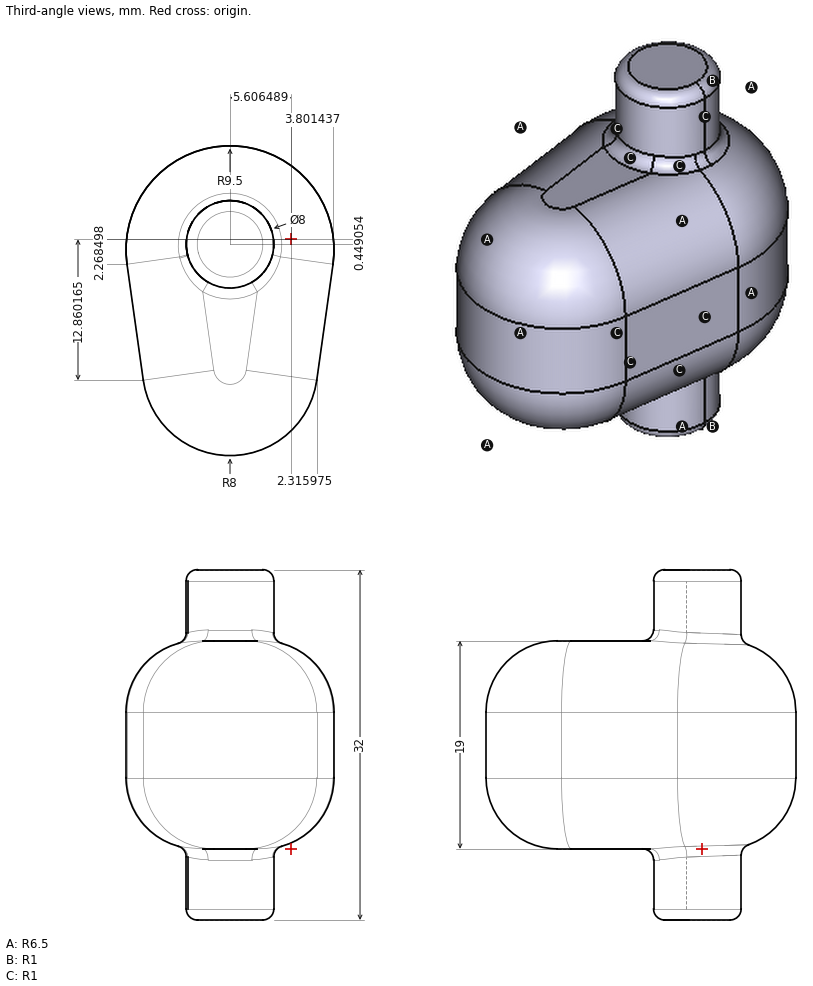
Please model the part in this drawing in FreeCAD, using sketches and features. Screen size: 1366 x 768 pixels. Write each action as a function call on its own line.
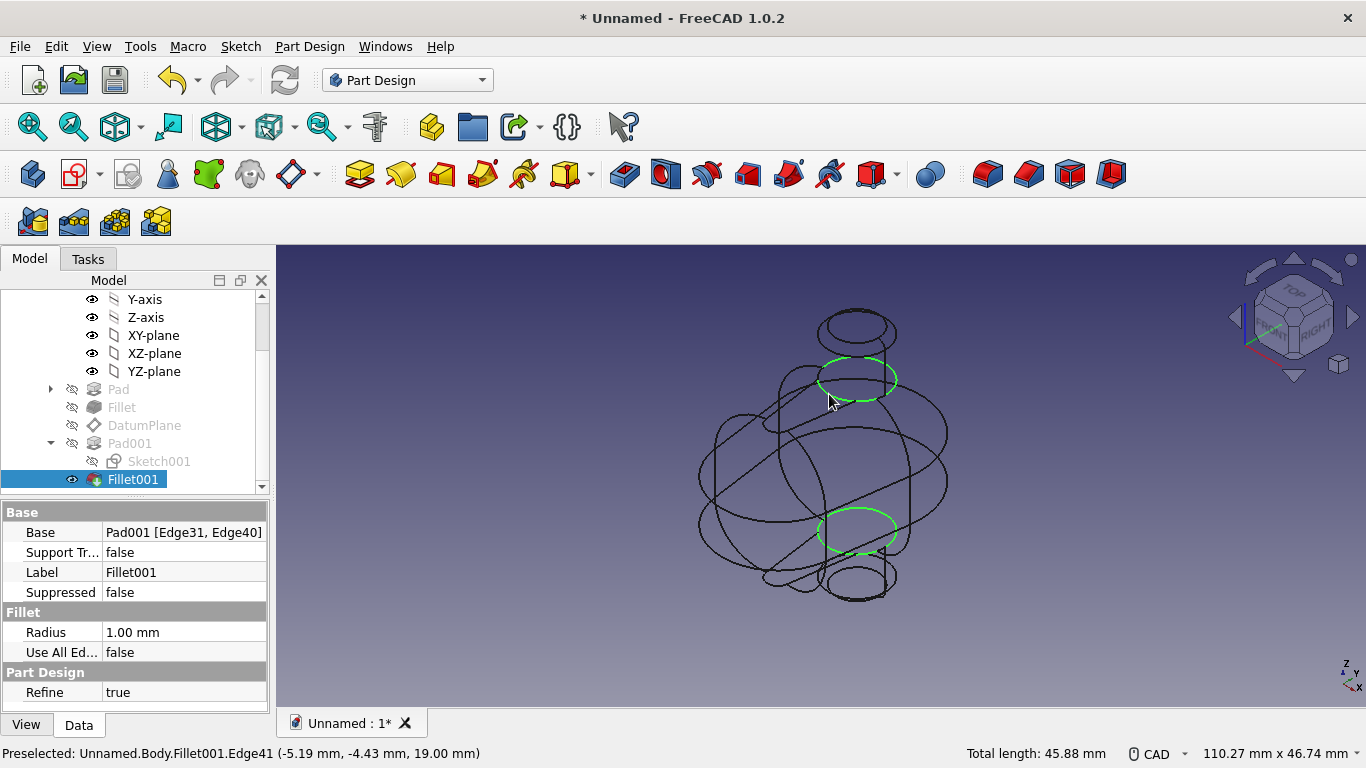
click(819, 372, ctrl)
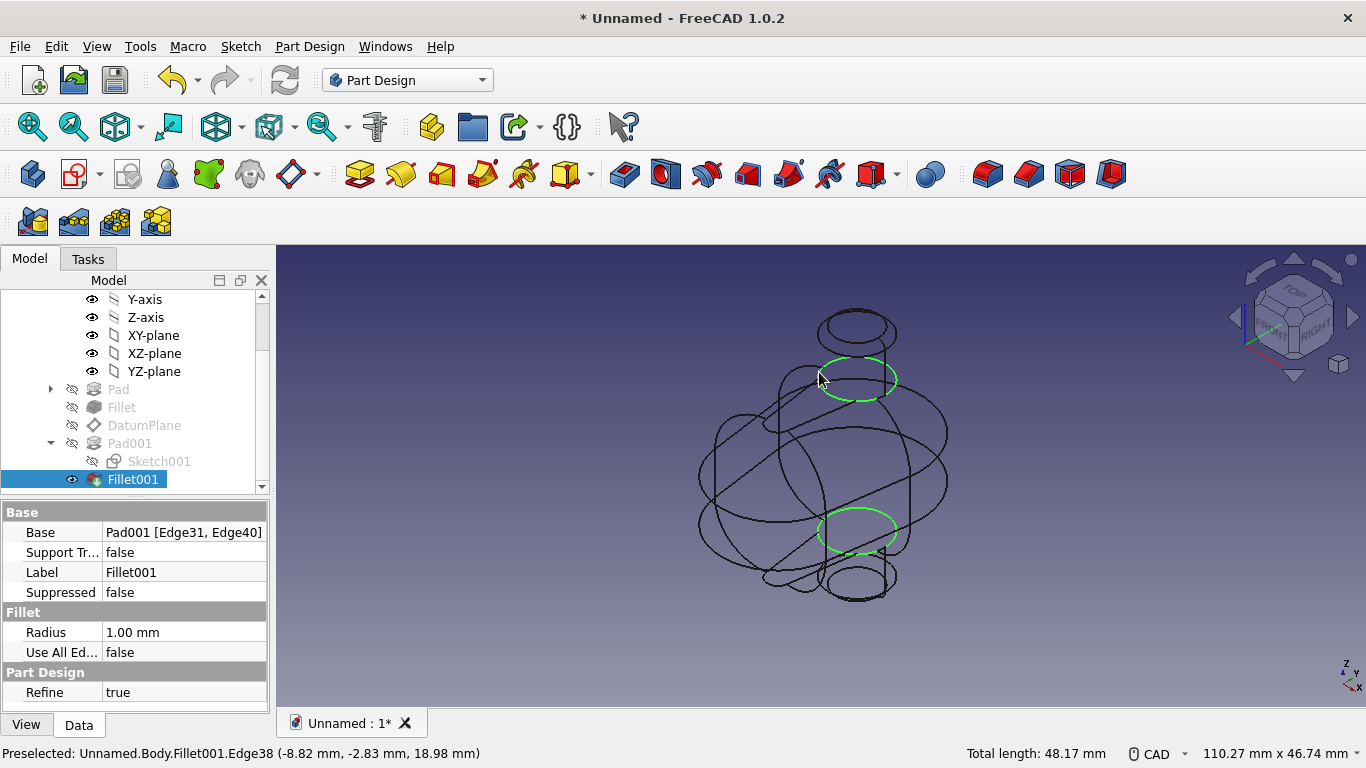
key(v)
key(1)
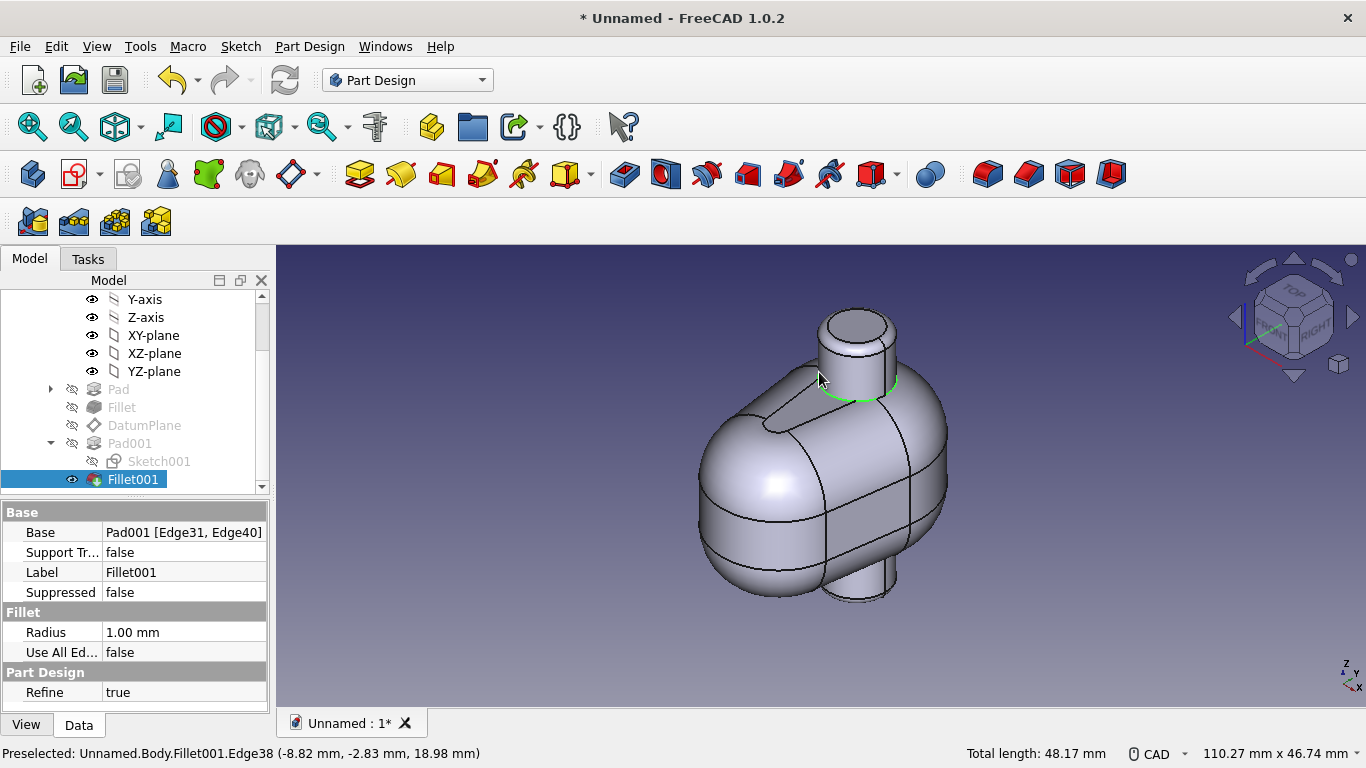
click(988, 174)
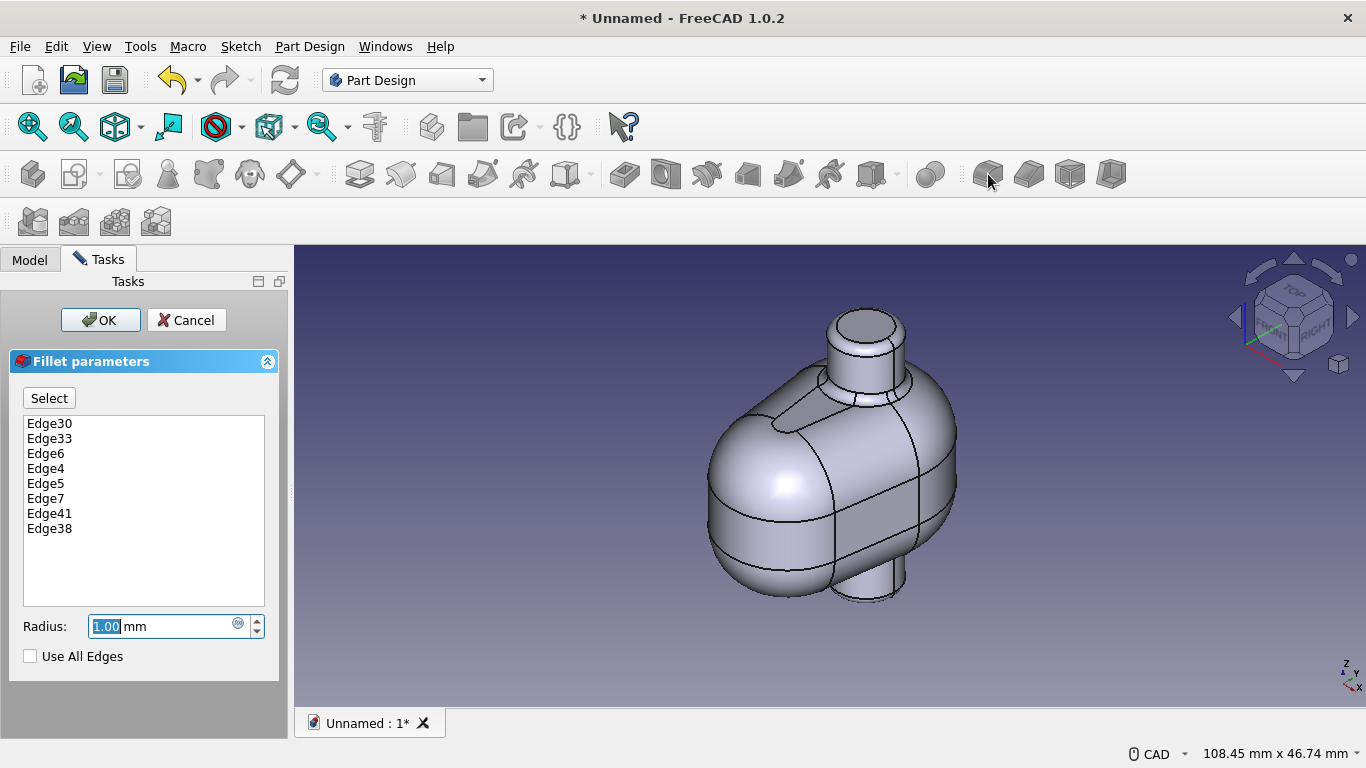
text(1)
key(Tab)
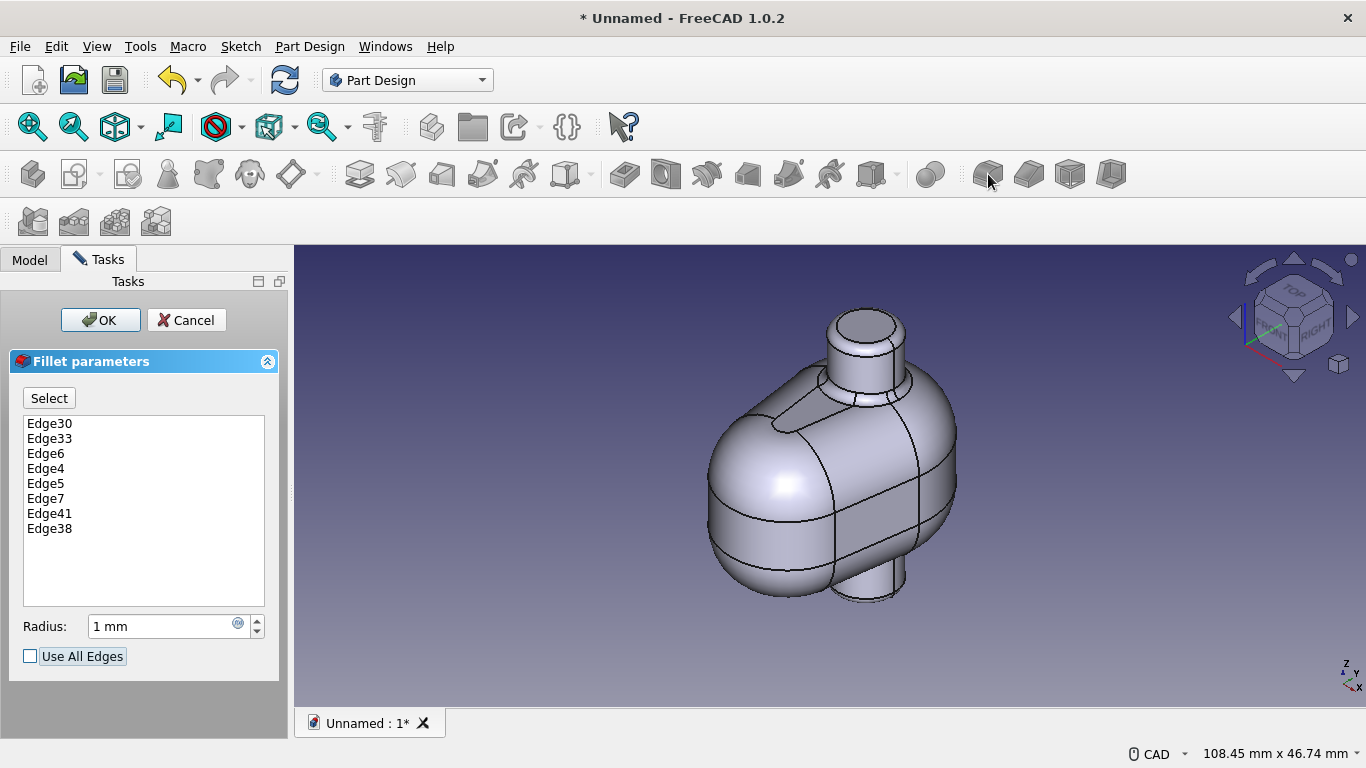
click(101, 320)